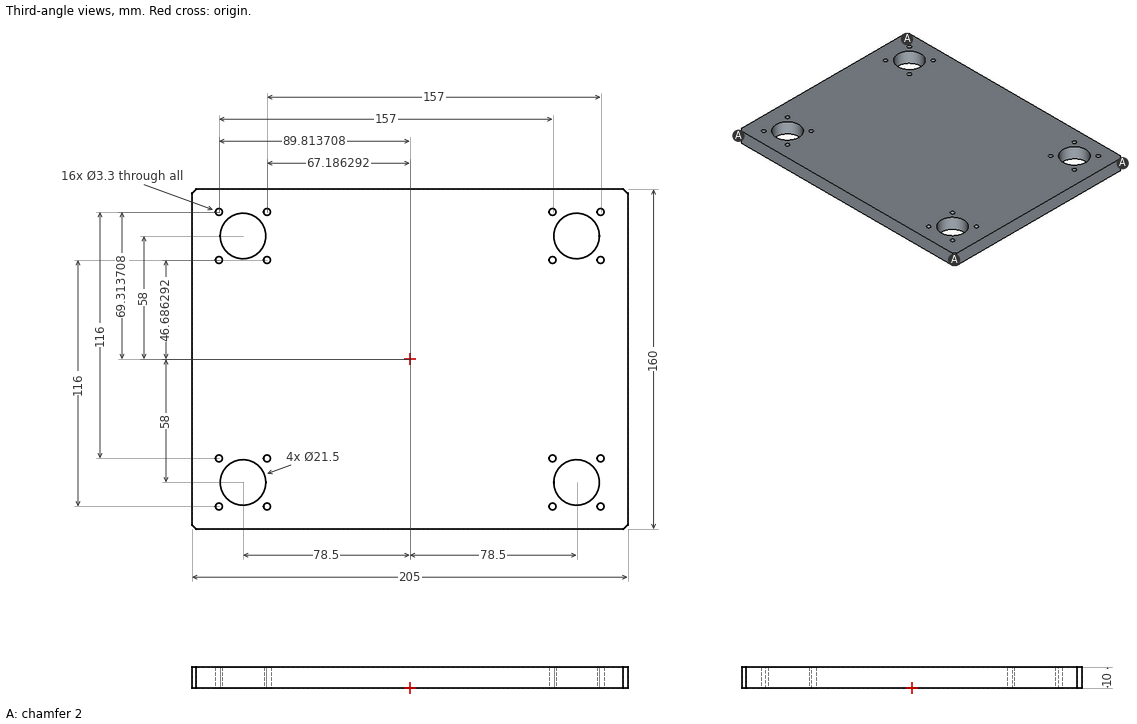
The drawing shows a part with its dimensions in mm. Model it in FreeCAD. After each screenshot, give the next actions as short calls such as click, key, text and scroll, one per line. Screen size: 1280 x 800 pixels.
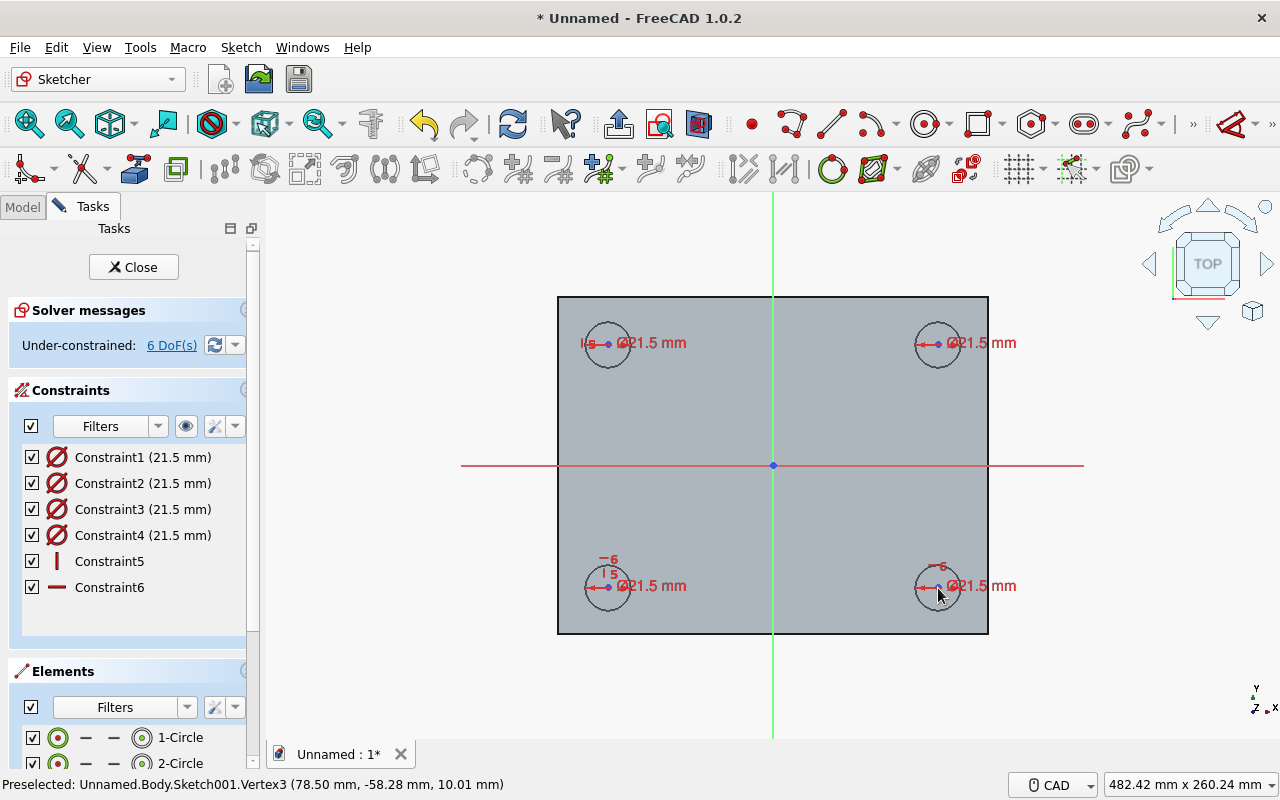
click(938, 588)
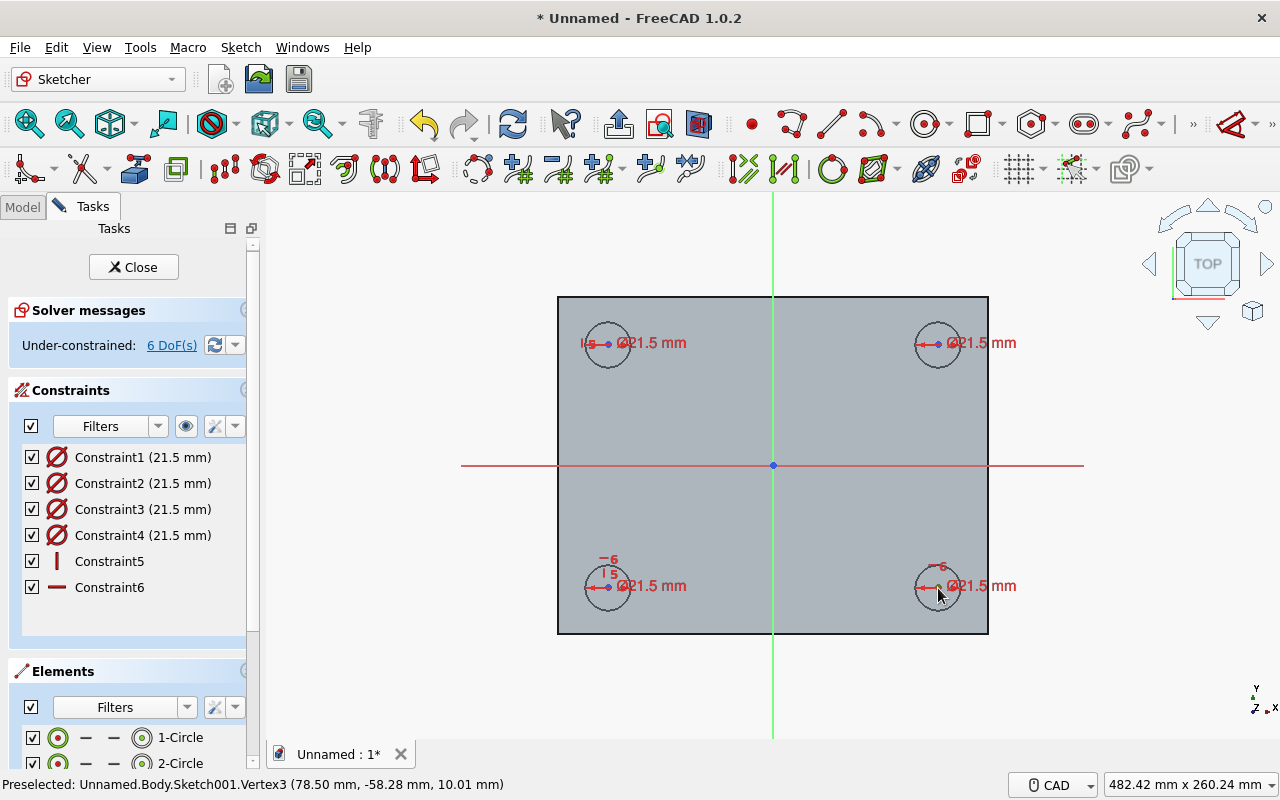
click(938, 345)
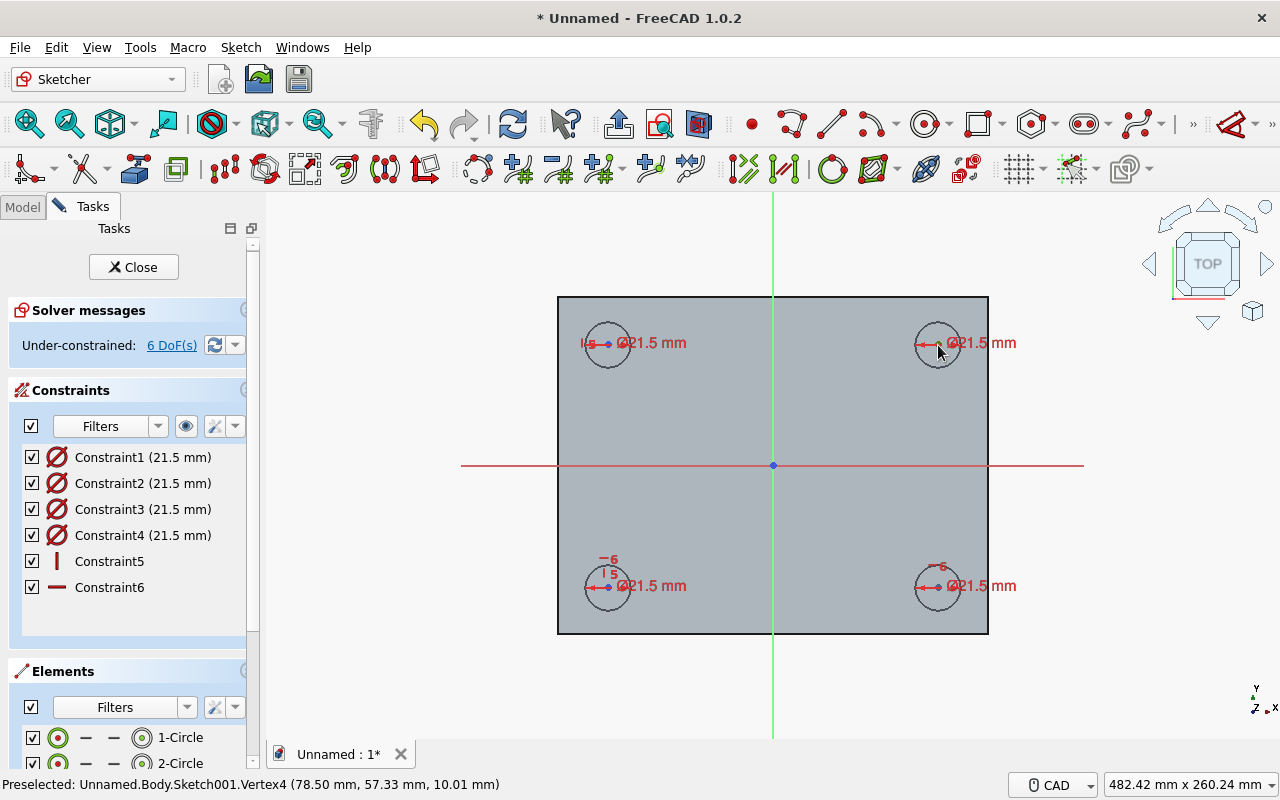
key(v)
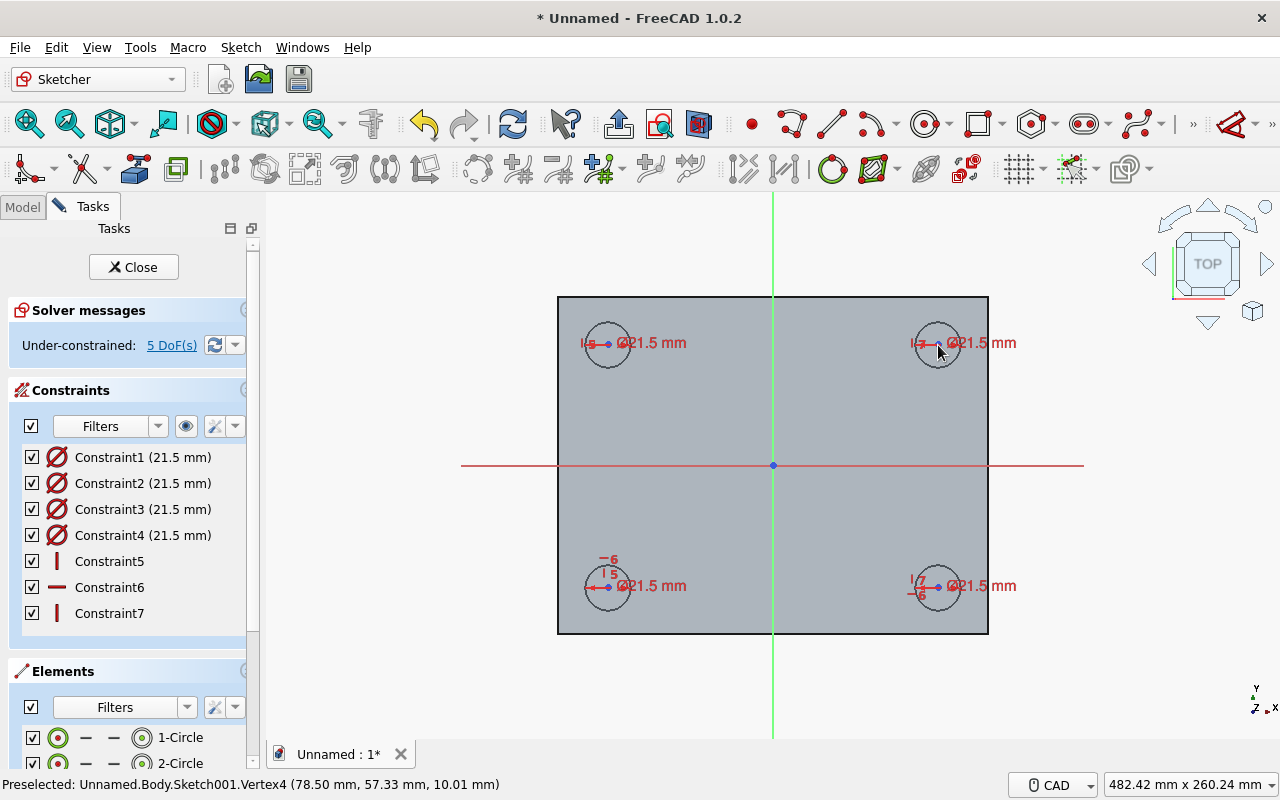
click(608, 345)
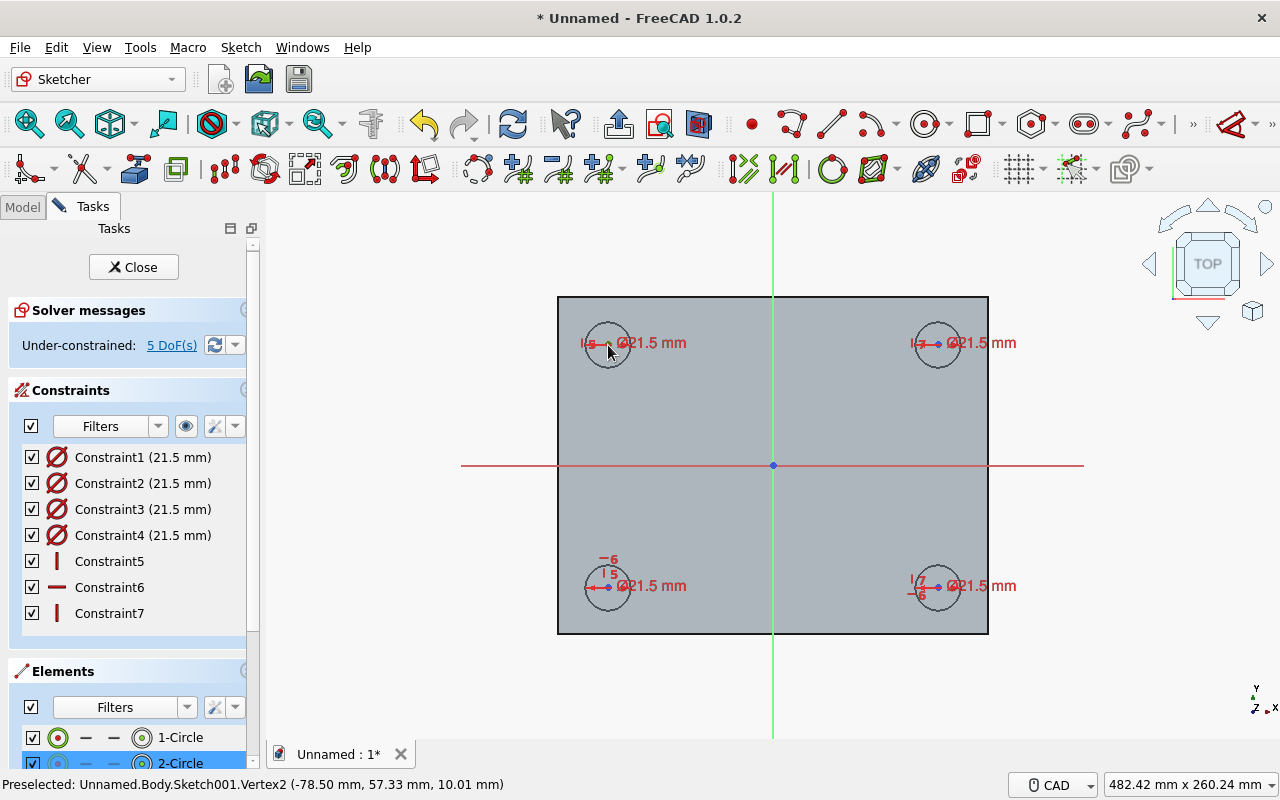
click(938, 345)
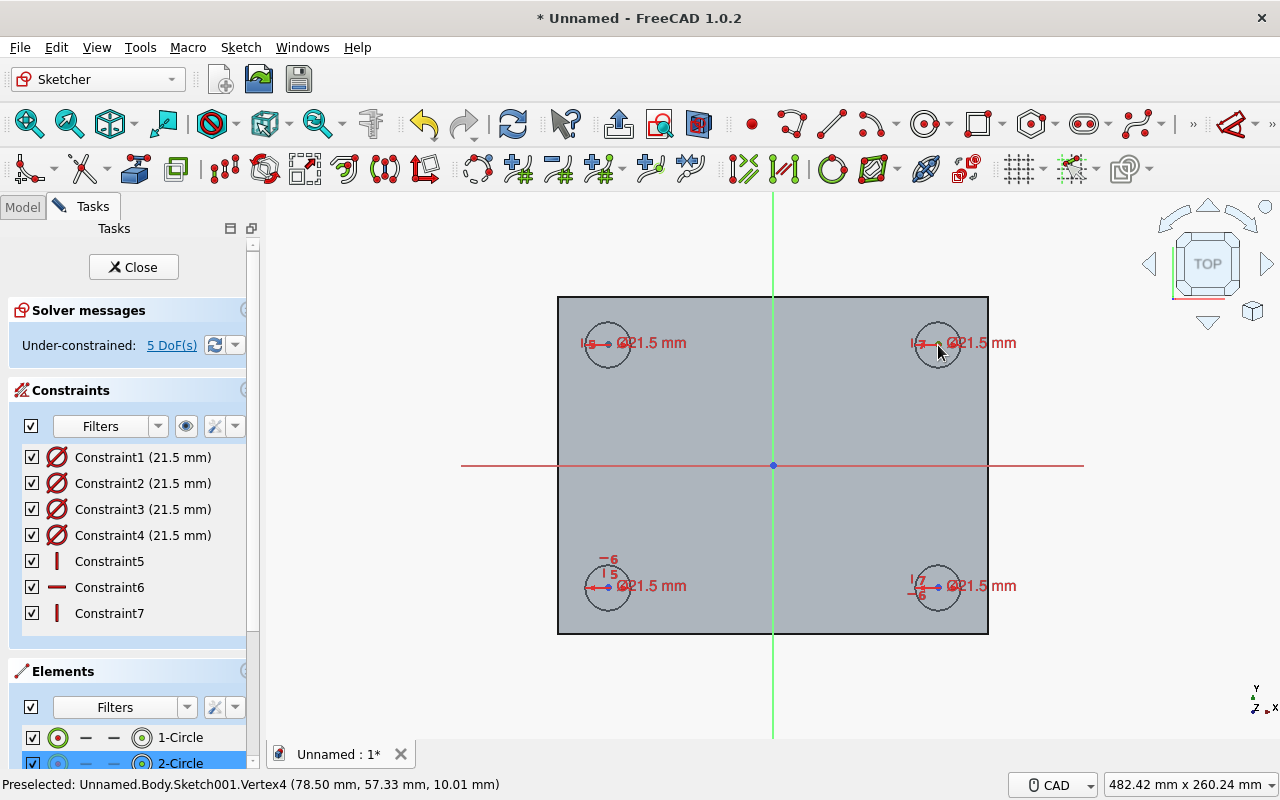
key(h)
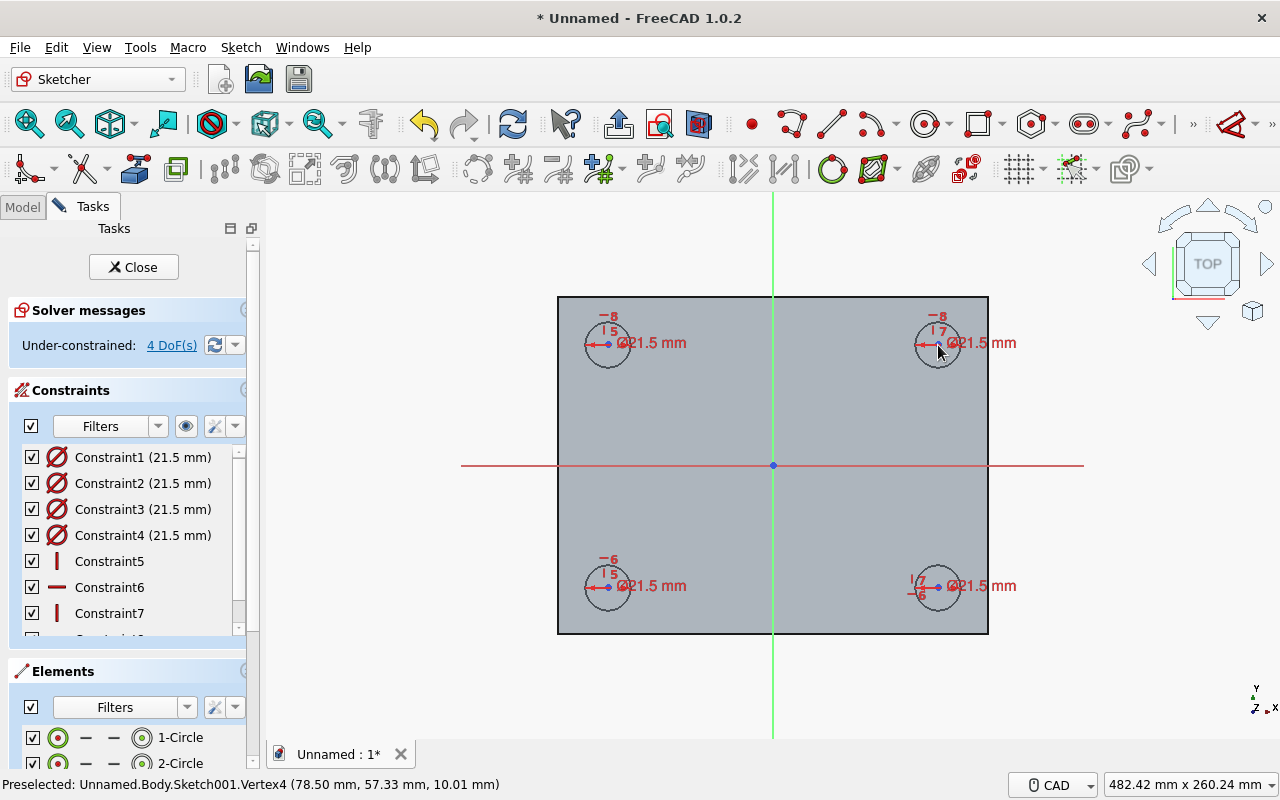
click(1232, 124)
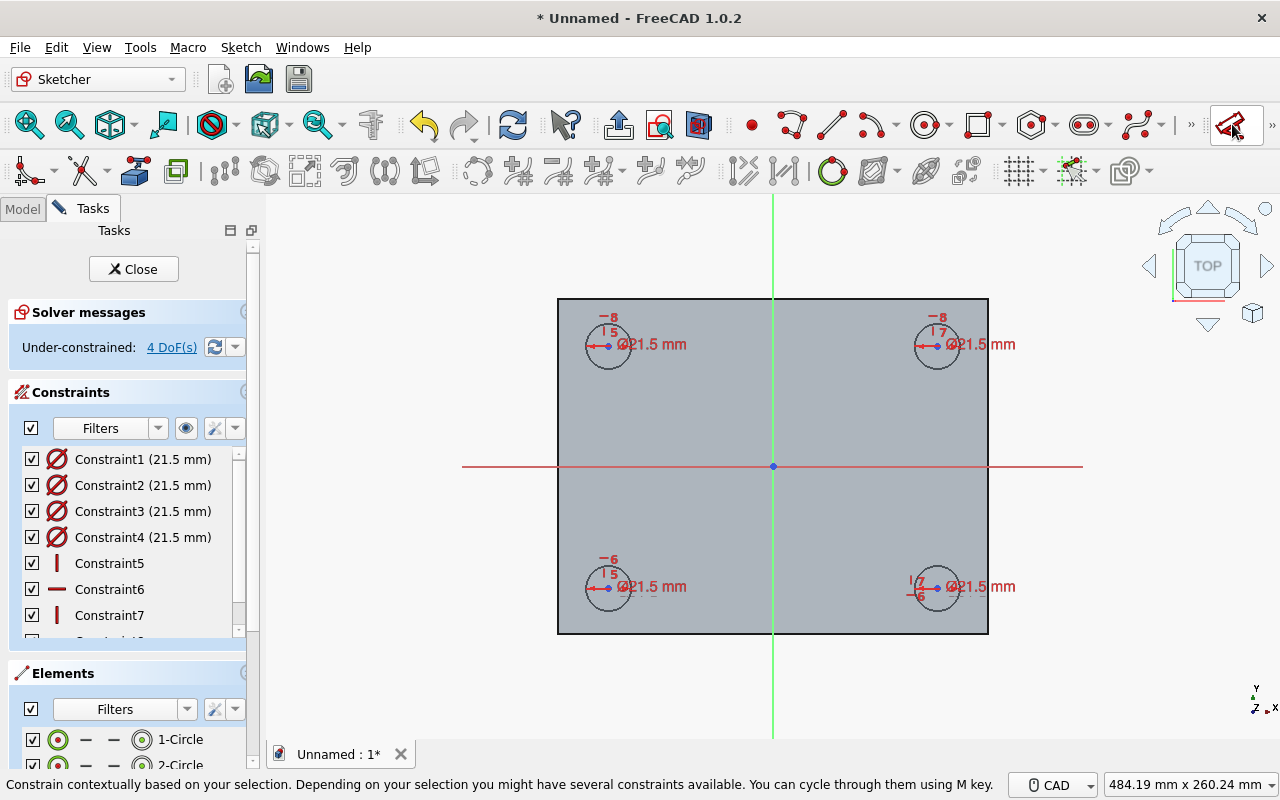
click(609, 589)
click(575, 528)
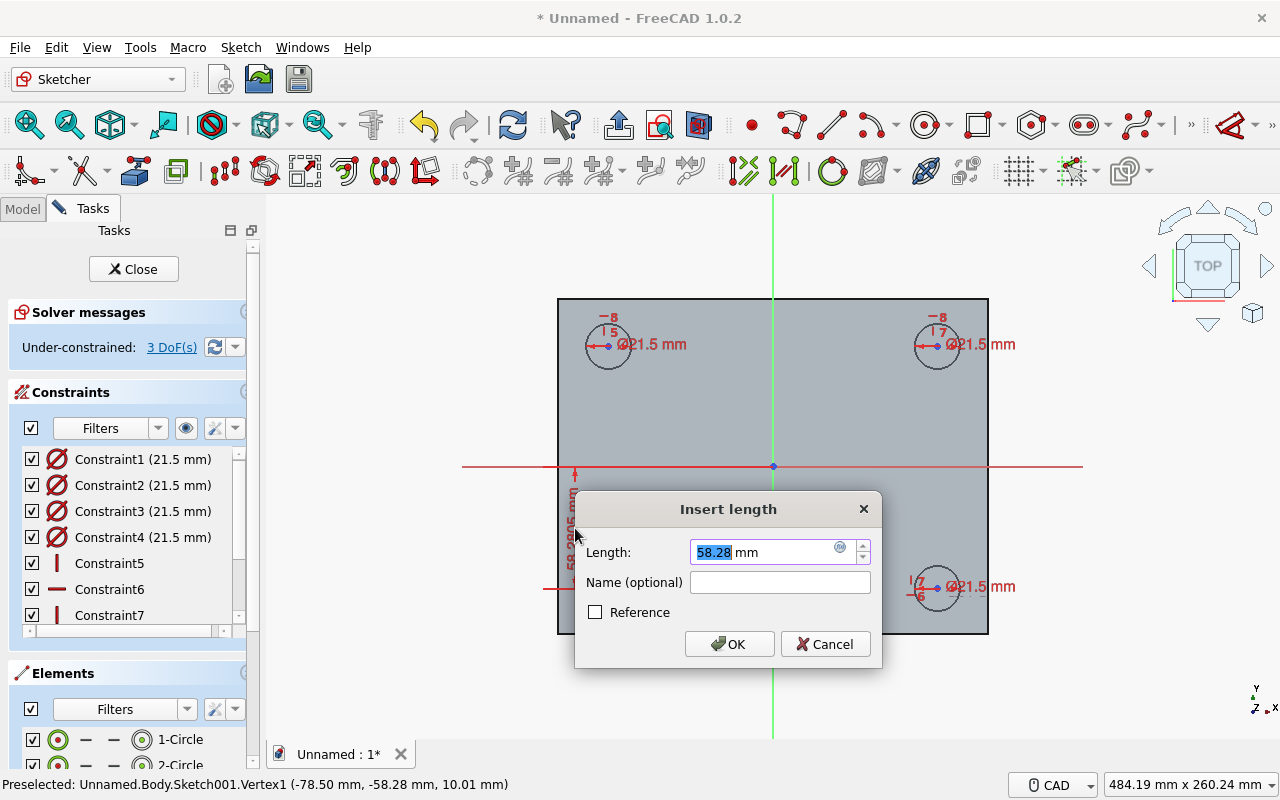
text(58)
key(Return)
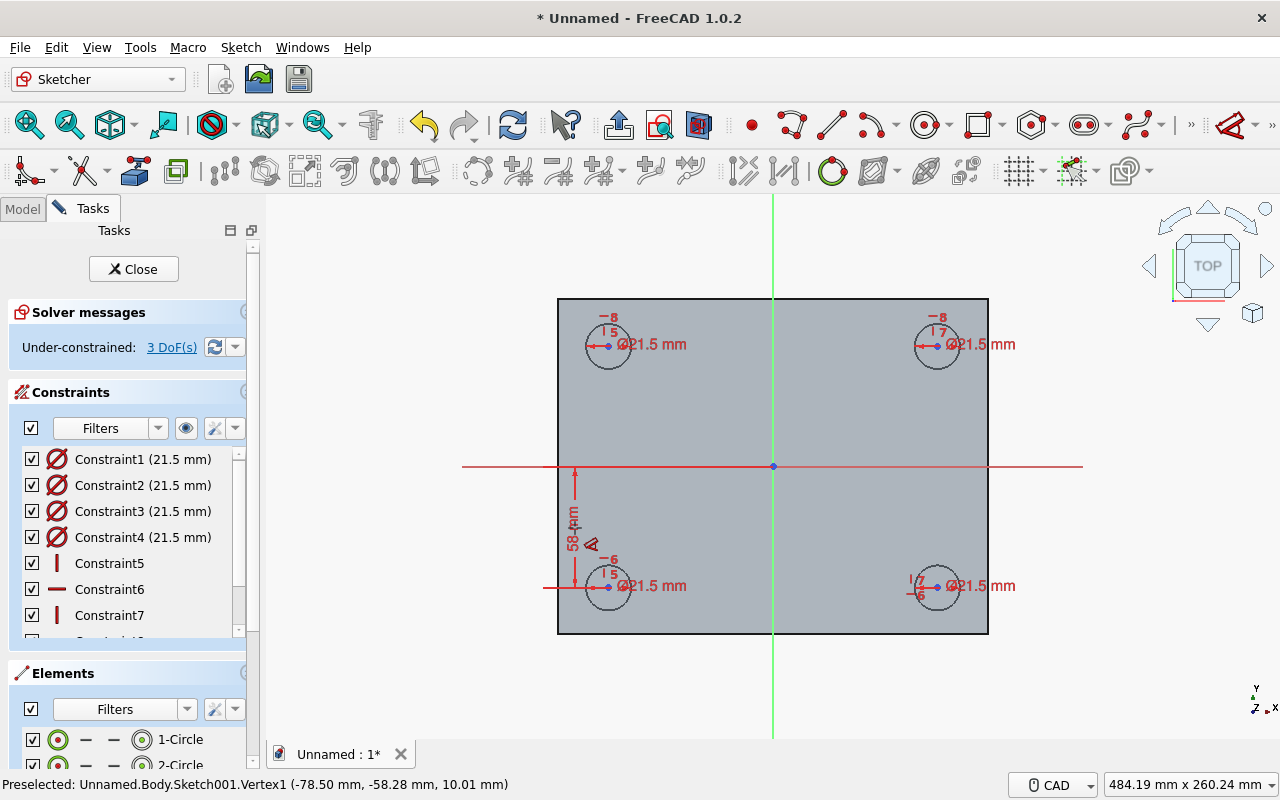
click(609, 346)
click(575, 406)